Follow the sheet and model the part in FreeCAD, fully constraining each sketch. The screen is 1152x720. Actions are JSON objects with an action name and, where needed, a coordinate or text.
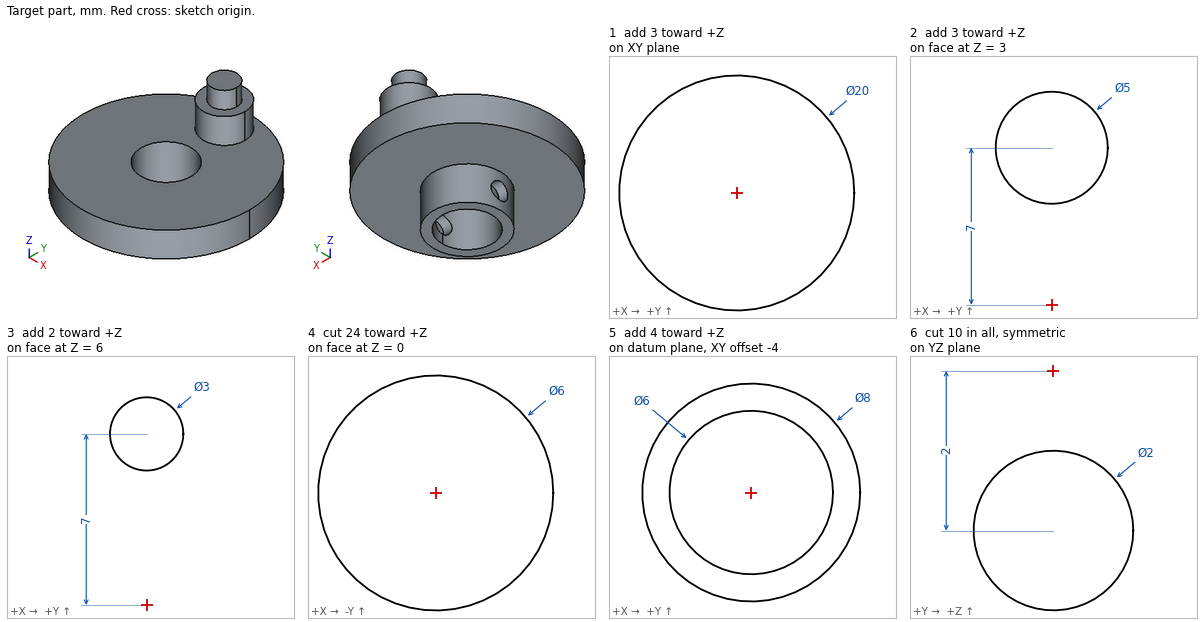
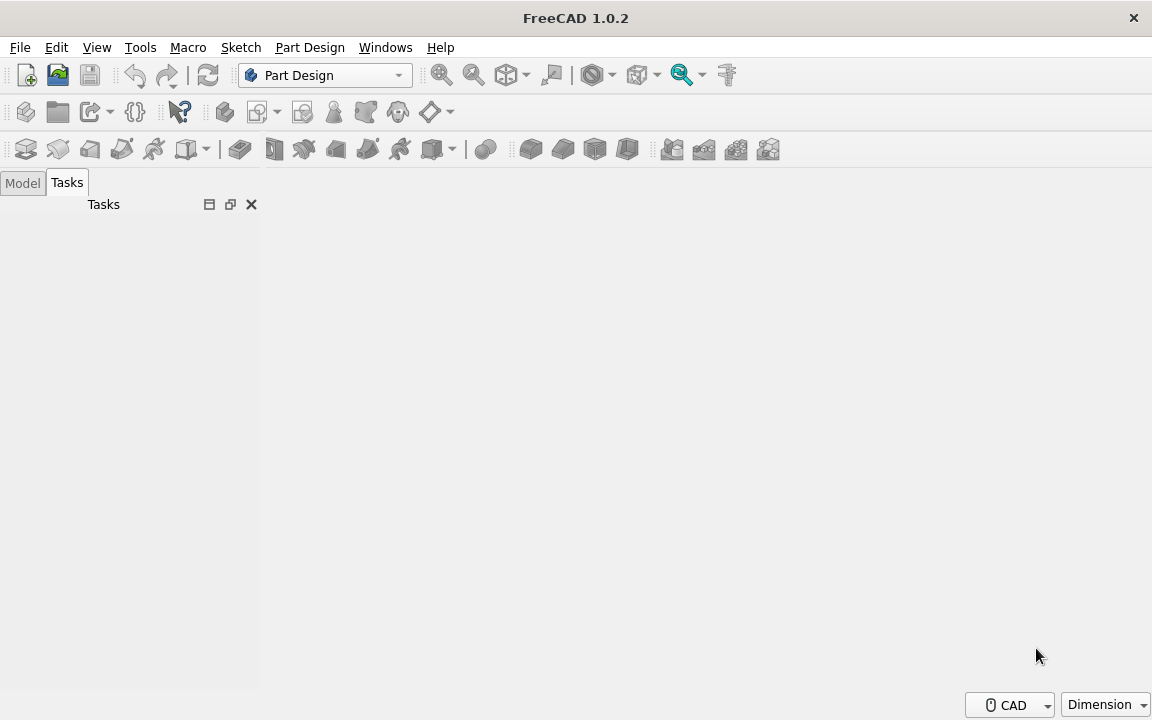
{"action": "left_click", "coordinate": [1016, 76]}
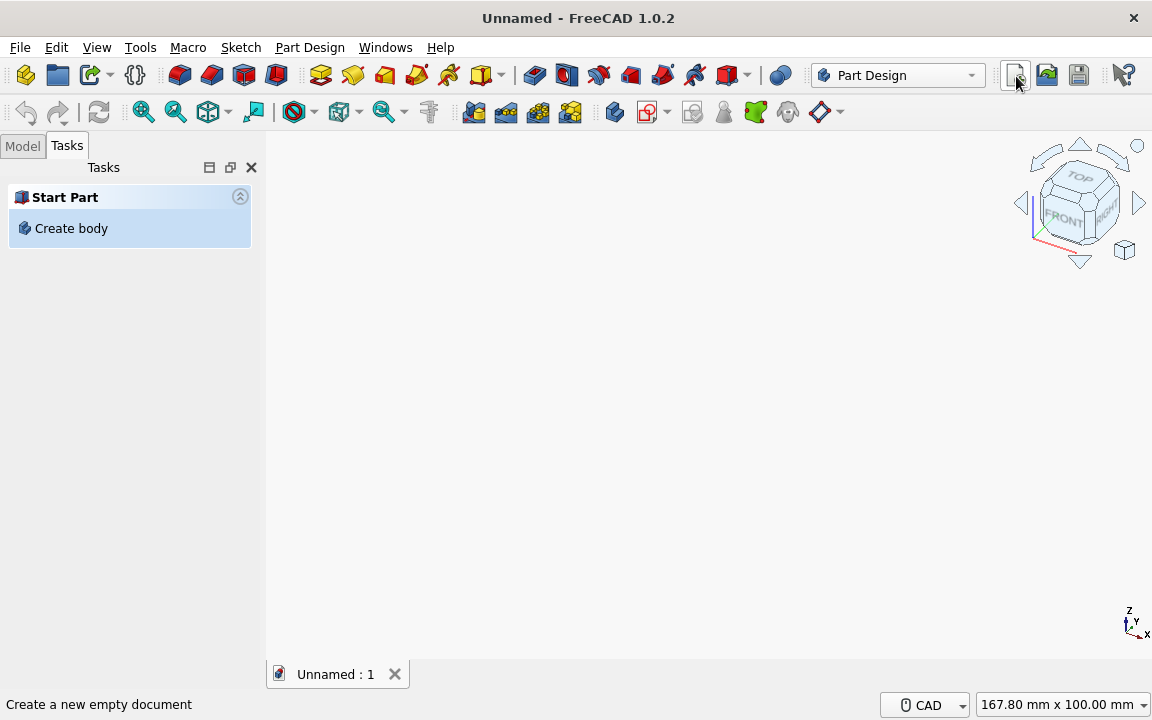
{"action": "left_click", "coordinate": [648, 112]}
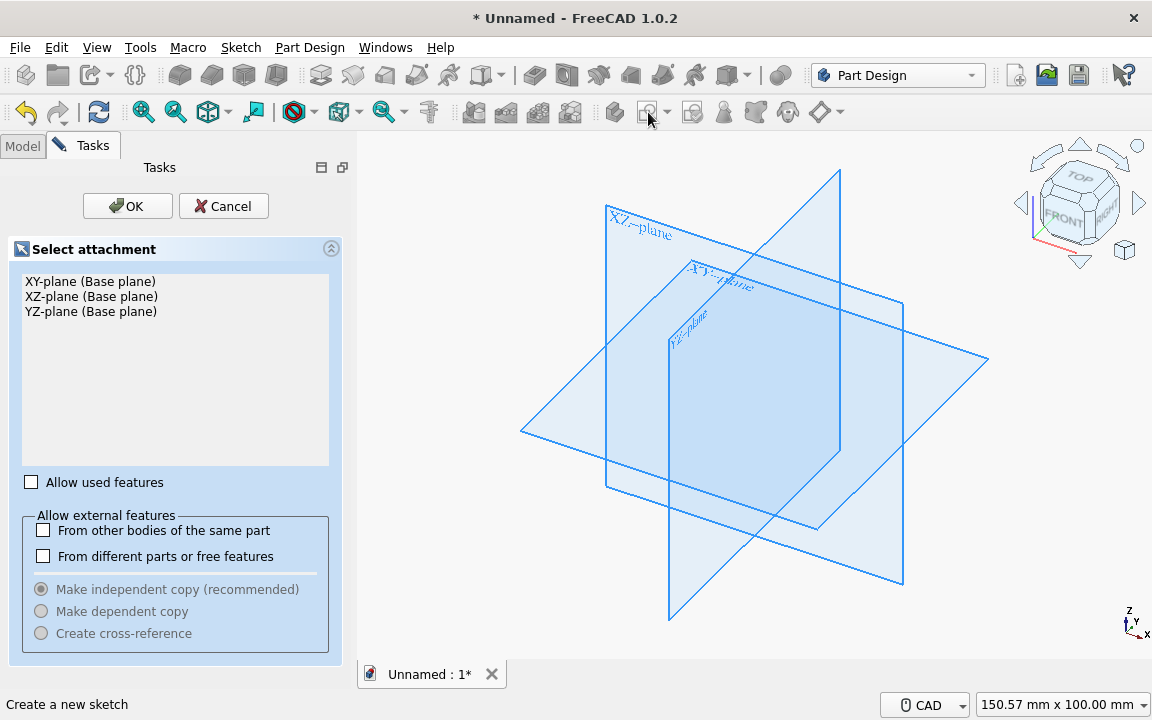
{"action": "left_click", "coordinate": [82, 282]}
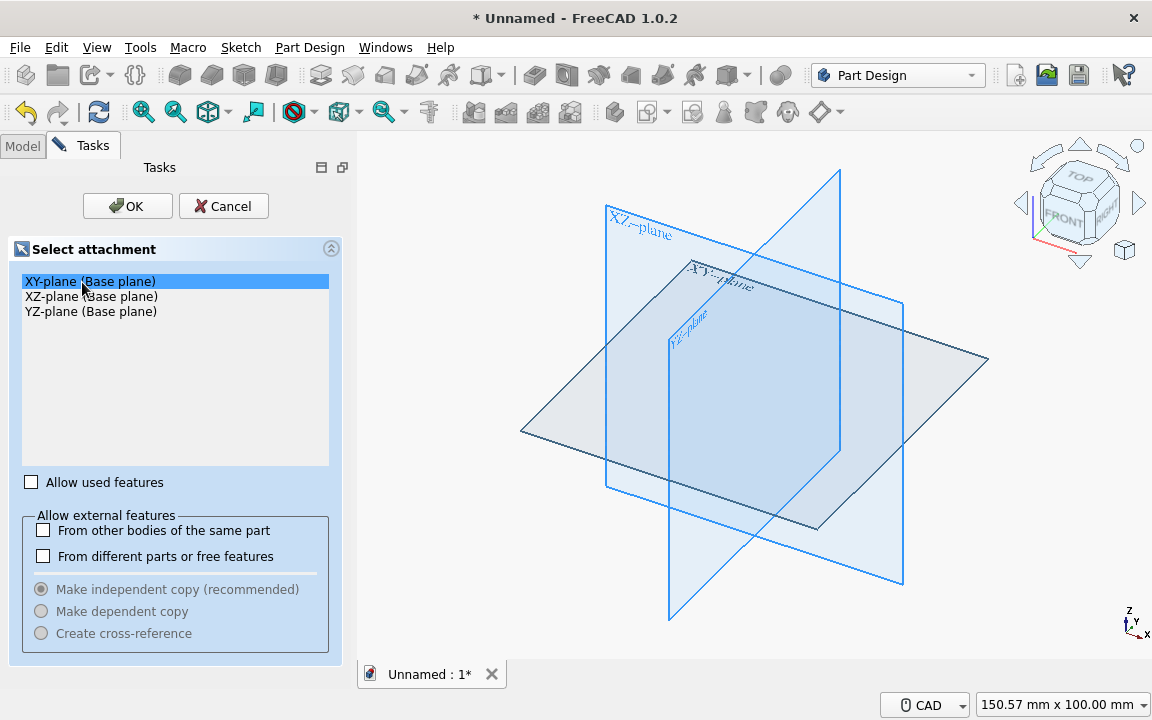
{"action": "left_click", "coordinate": [128, 206]}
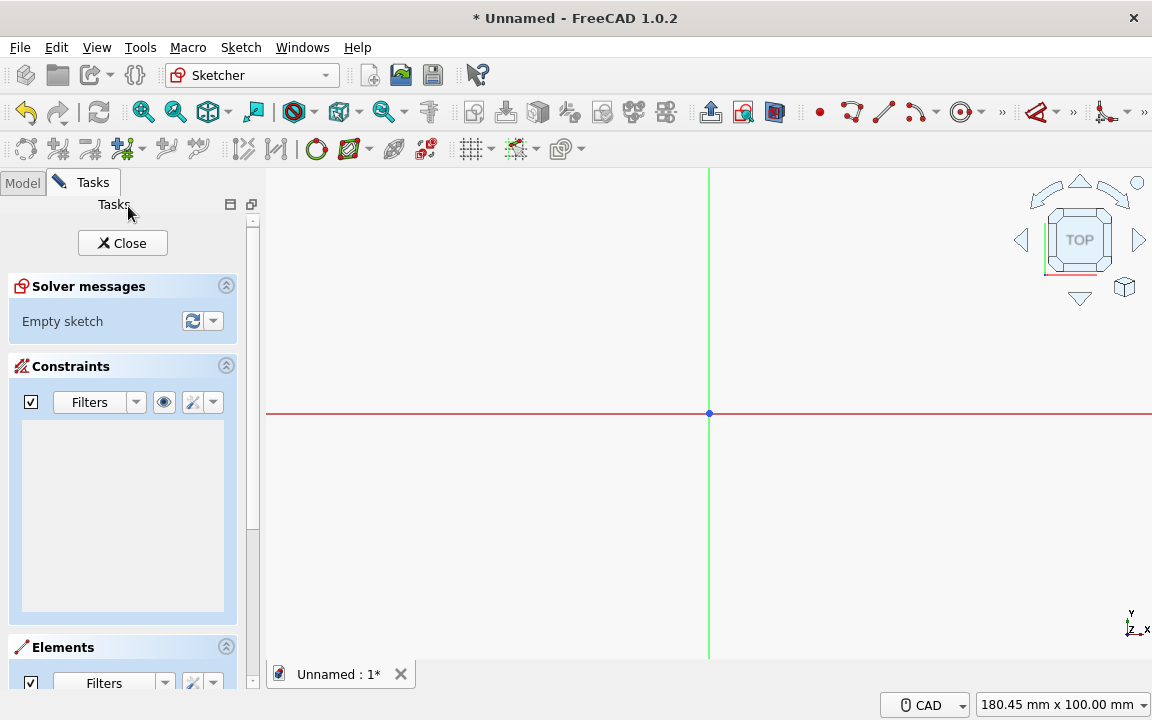
{"action": "scroll", "coordinate": [739, 414], "scroll_direction": "up", "scroll_amount": 6}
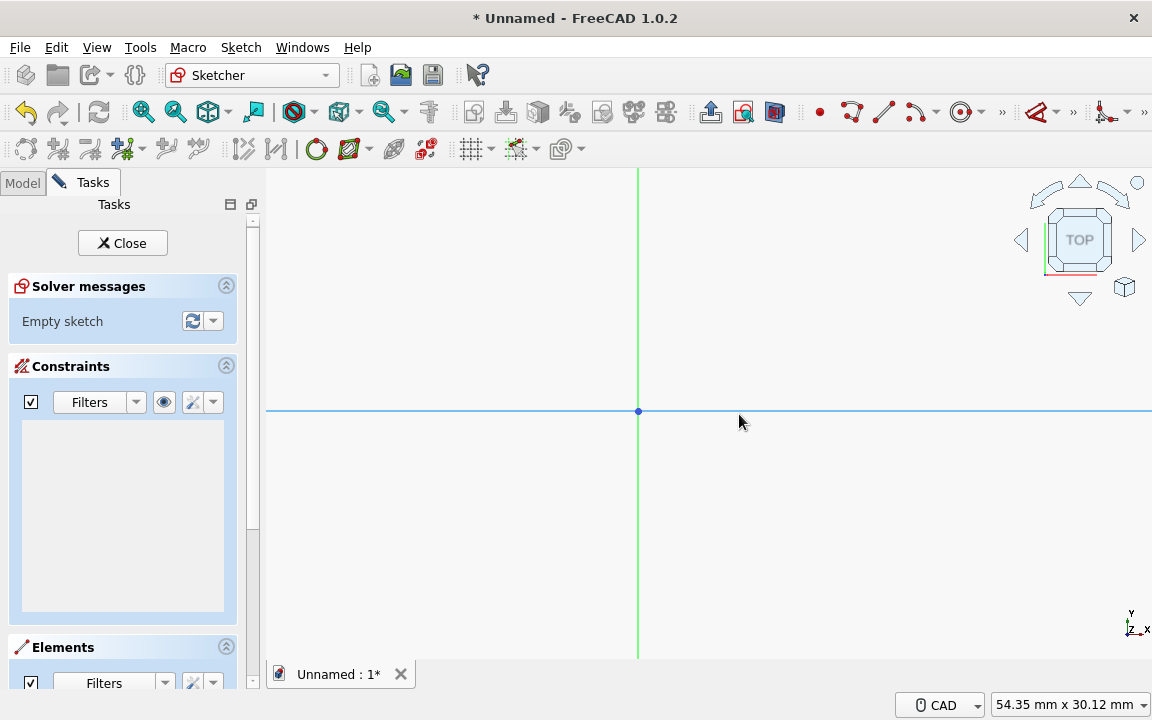
{"action": "left_click", "coordinate": [962, 112]}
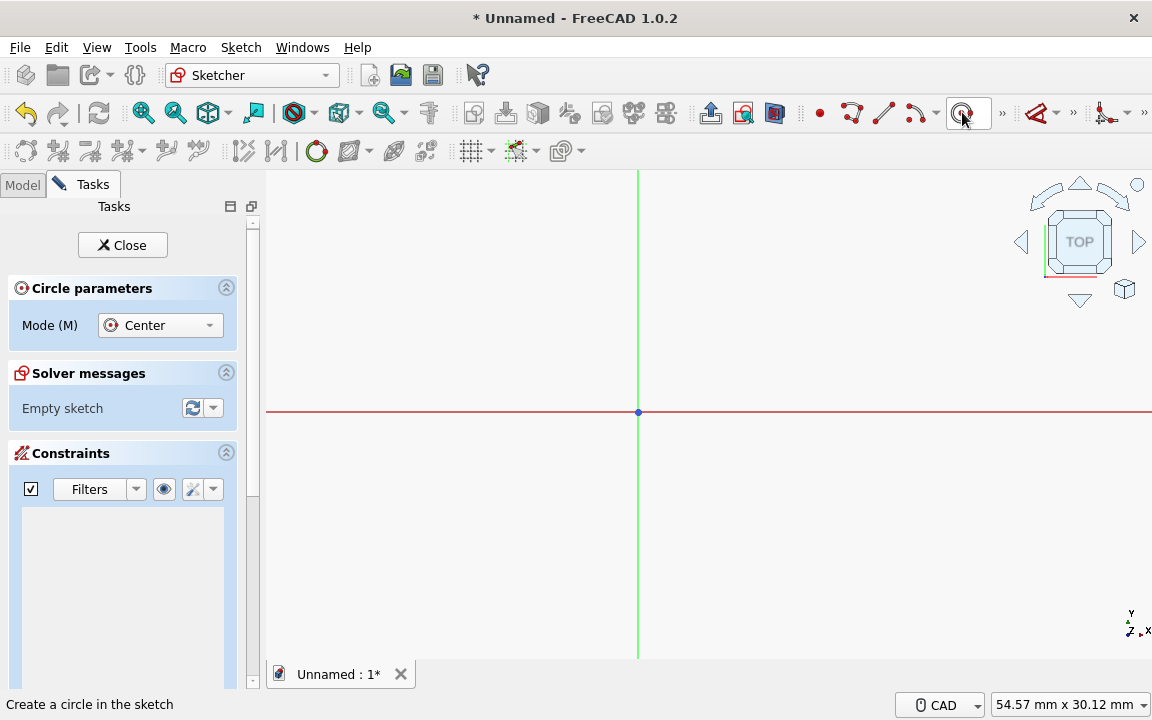
{"action": "left_click", "coordinate": [638, 412]}
{"action": "left_click", "coordinate": [753, 297]}
{"action": "key", "text": "Escape"}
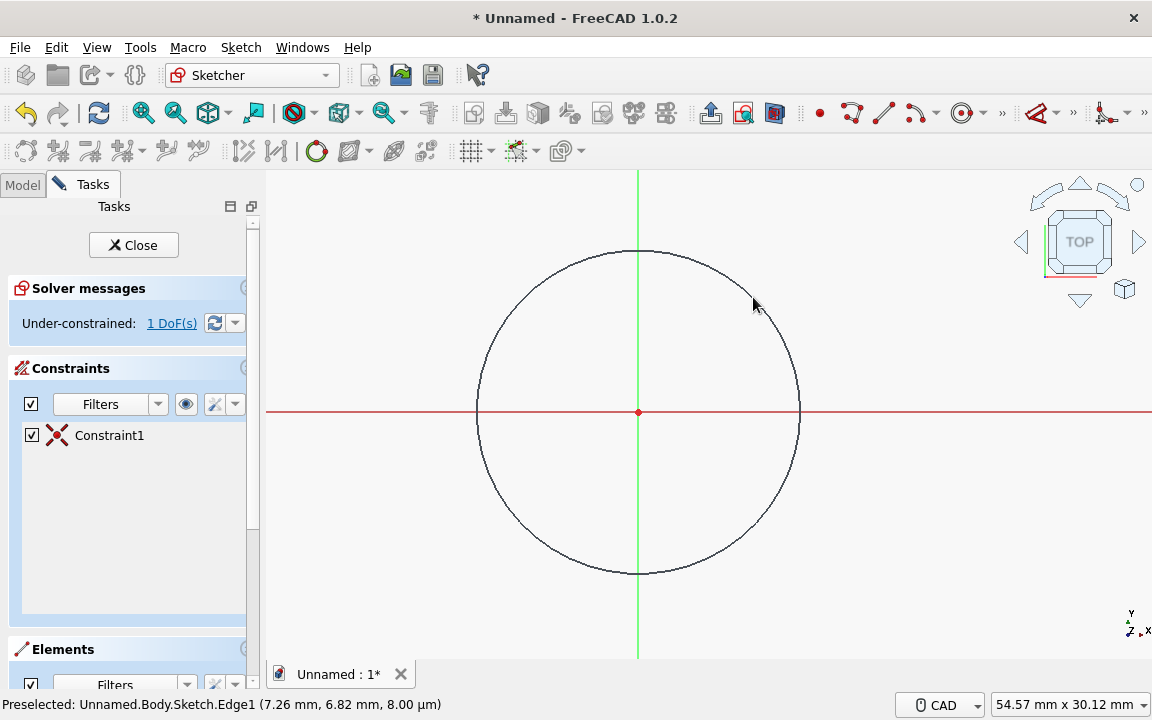
{"action": "left_click", "coordinate": [1036, 114]}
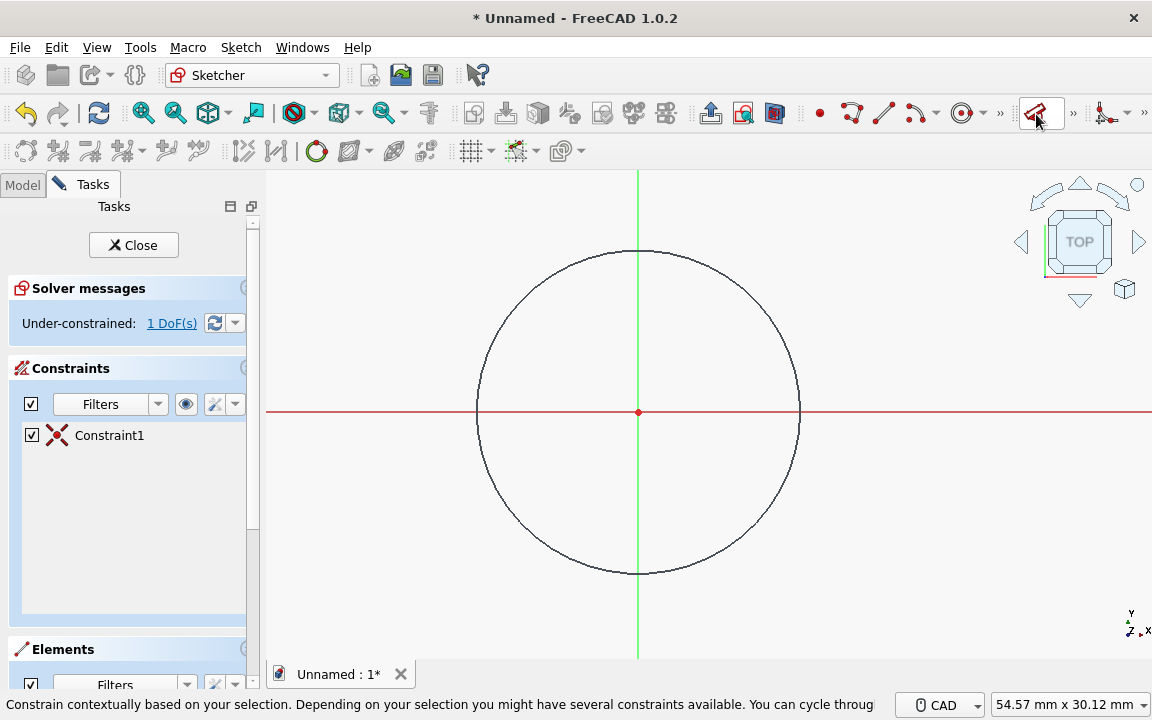
{"action": "left_click", "coordinate": [752, 297]}
{"action": "left_click", "coordinate": [774, 274]}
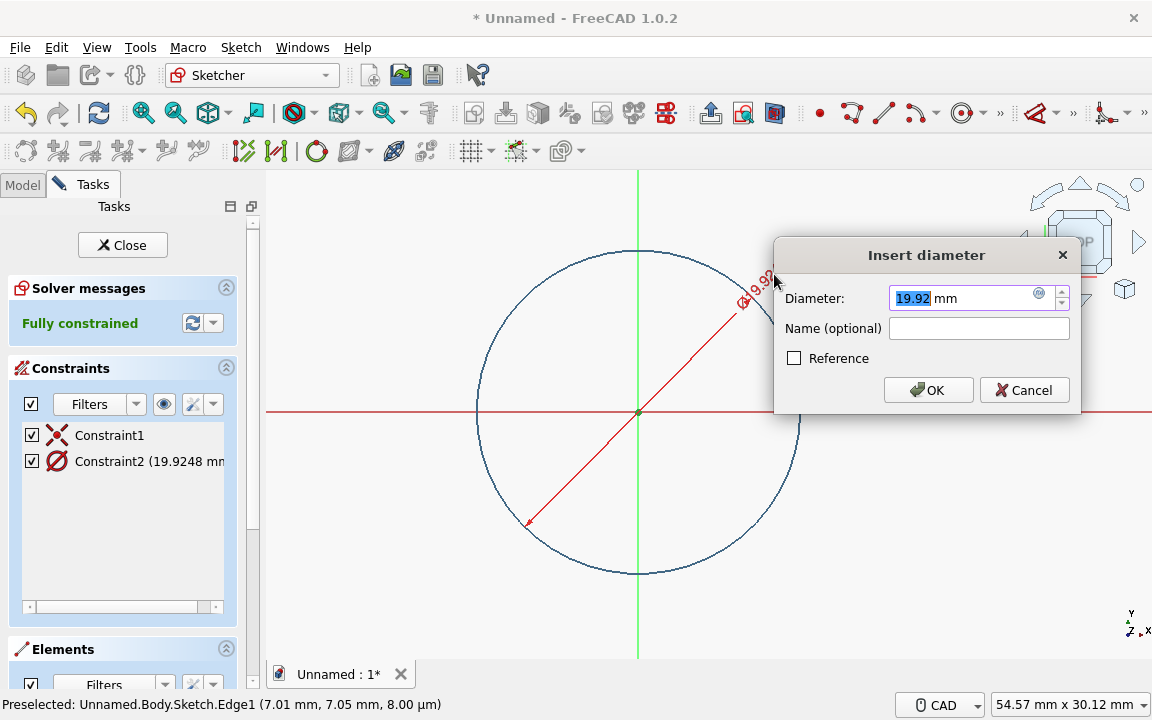
{"action": "type", "text": "20"}
{"action": "key", "text": "Return"}
{"action": "key", "text": "Escape"}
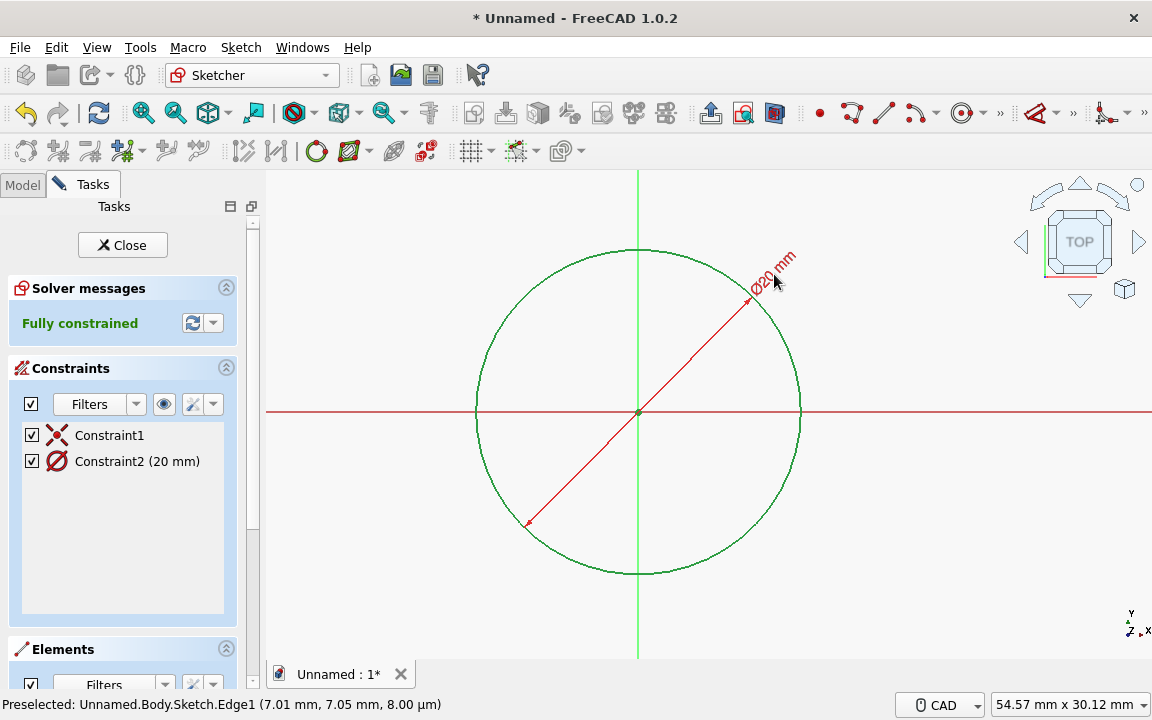
{"action": "left_click", "coordinate": [123, 245]}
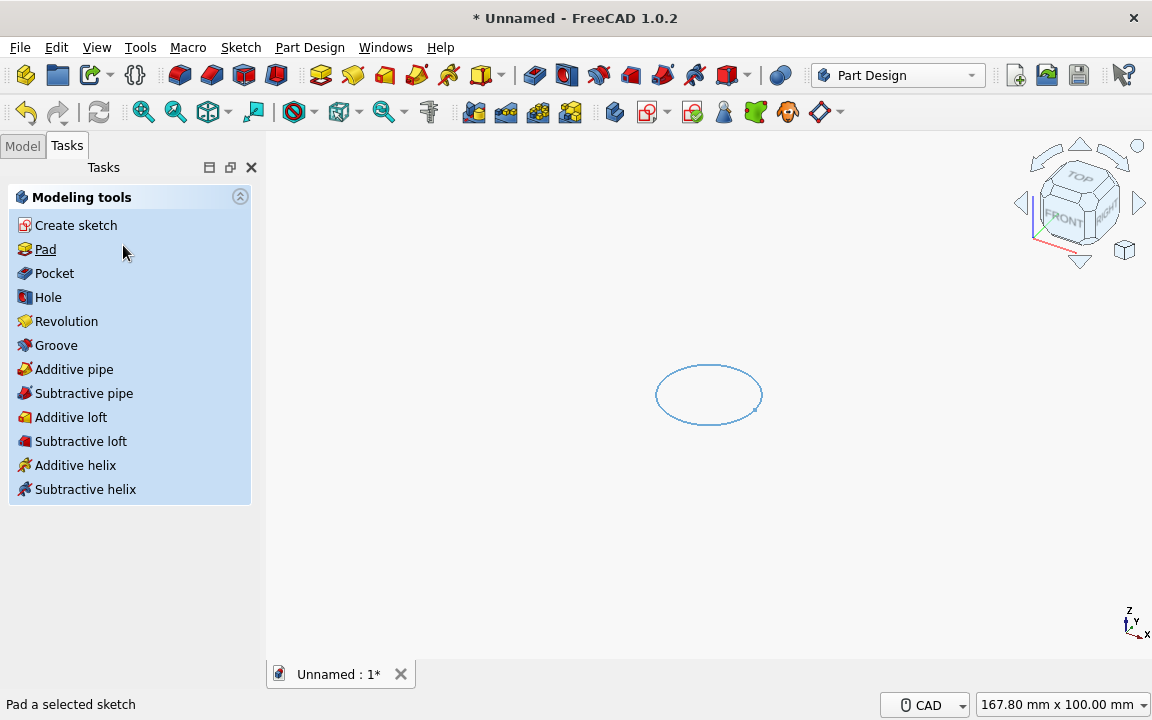
{"action": "left_click", "coordinate": [322, 76]}